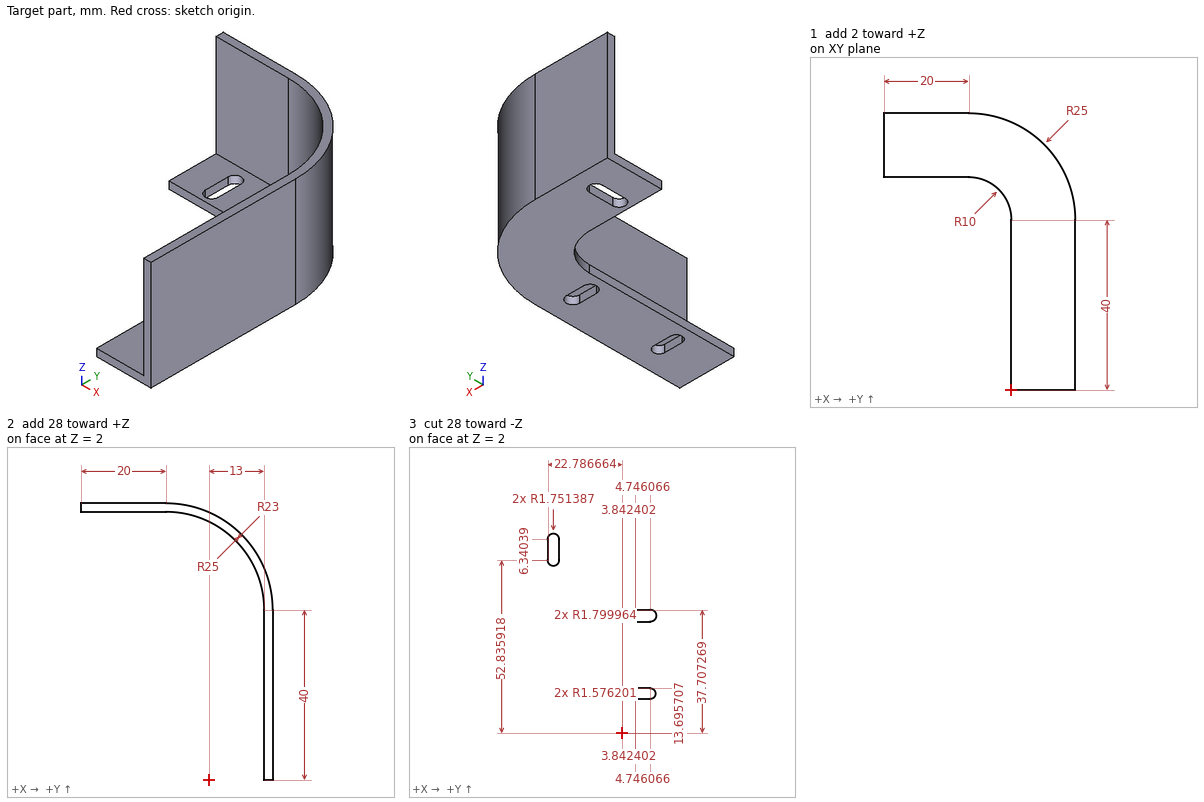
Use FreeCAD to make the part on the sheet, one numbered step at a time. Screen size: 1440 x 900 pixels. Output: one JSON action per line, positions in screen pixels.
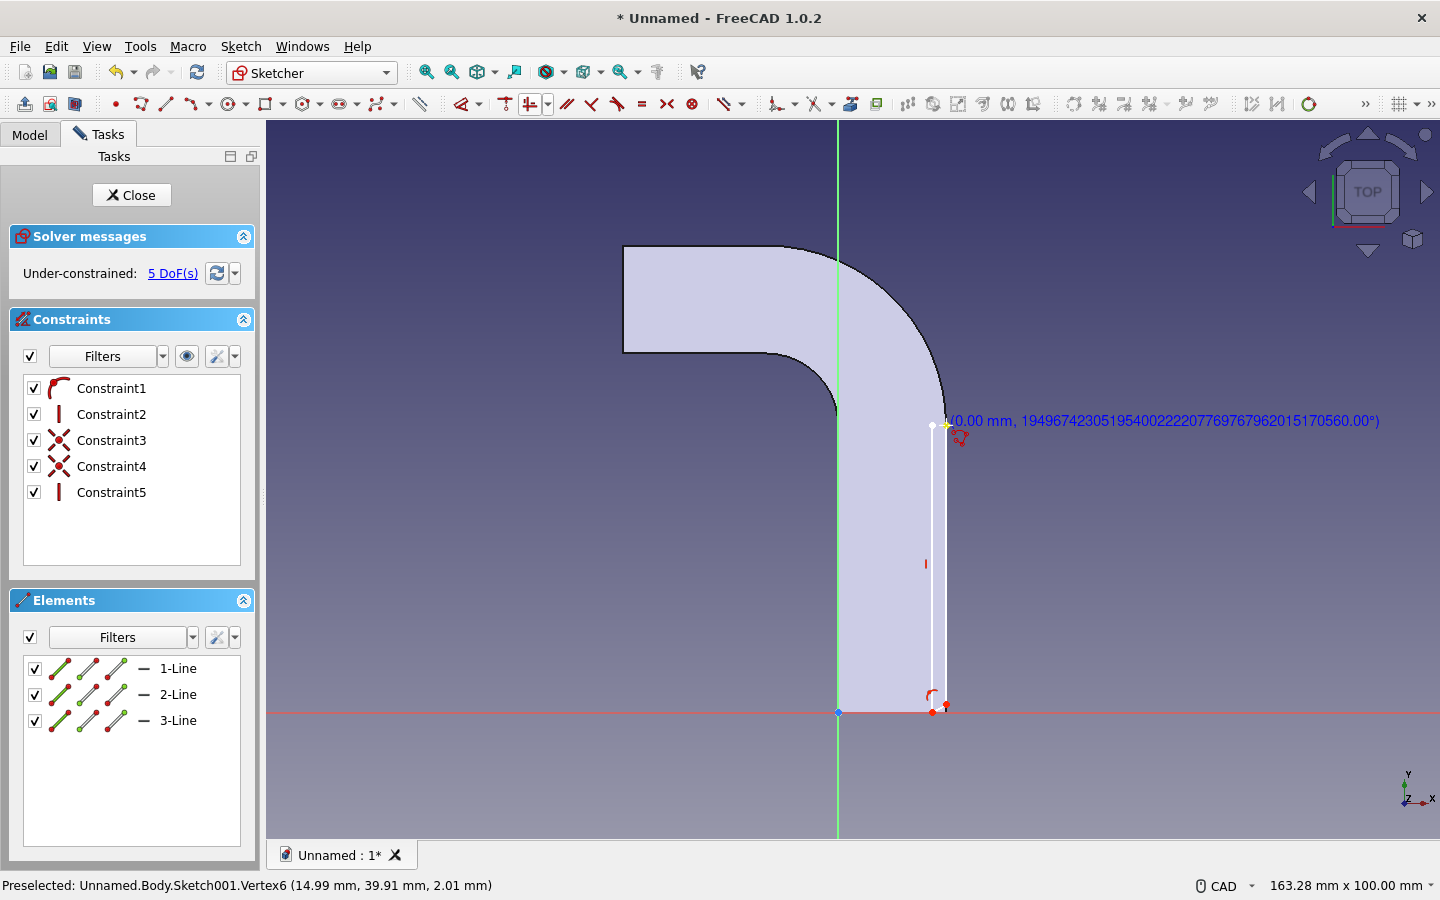
{"action": "left_click", "coordinate": [766, 246]}
{"action": "left_click", "coordinate": [623, 246]}
{"action": "left_click", "coordinate": [623, 260]}
{"action": "left_click", "coordinate": [766, 260]}
{"action": "right_click", "coordinate": [766, 260]}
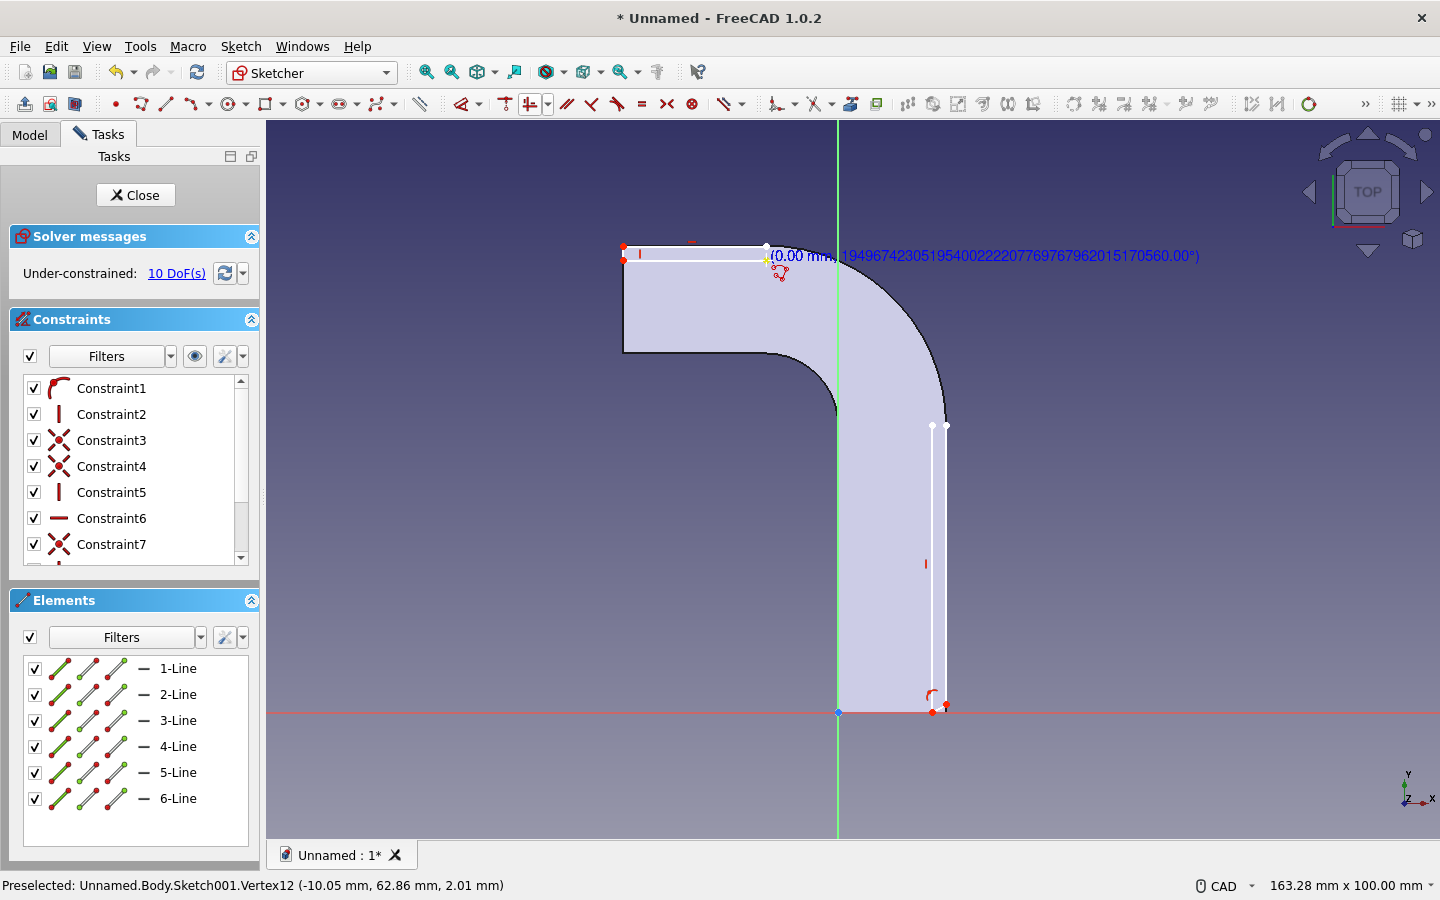
{"action": "left_click", "coordinate": [190, 104]}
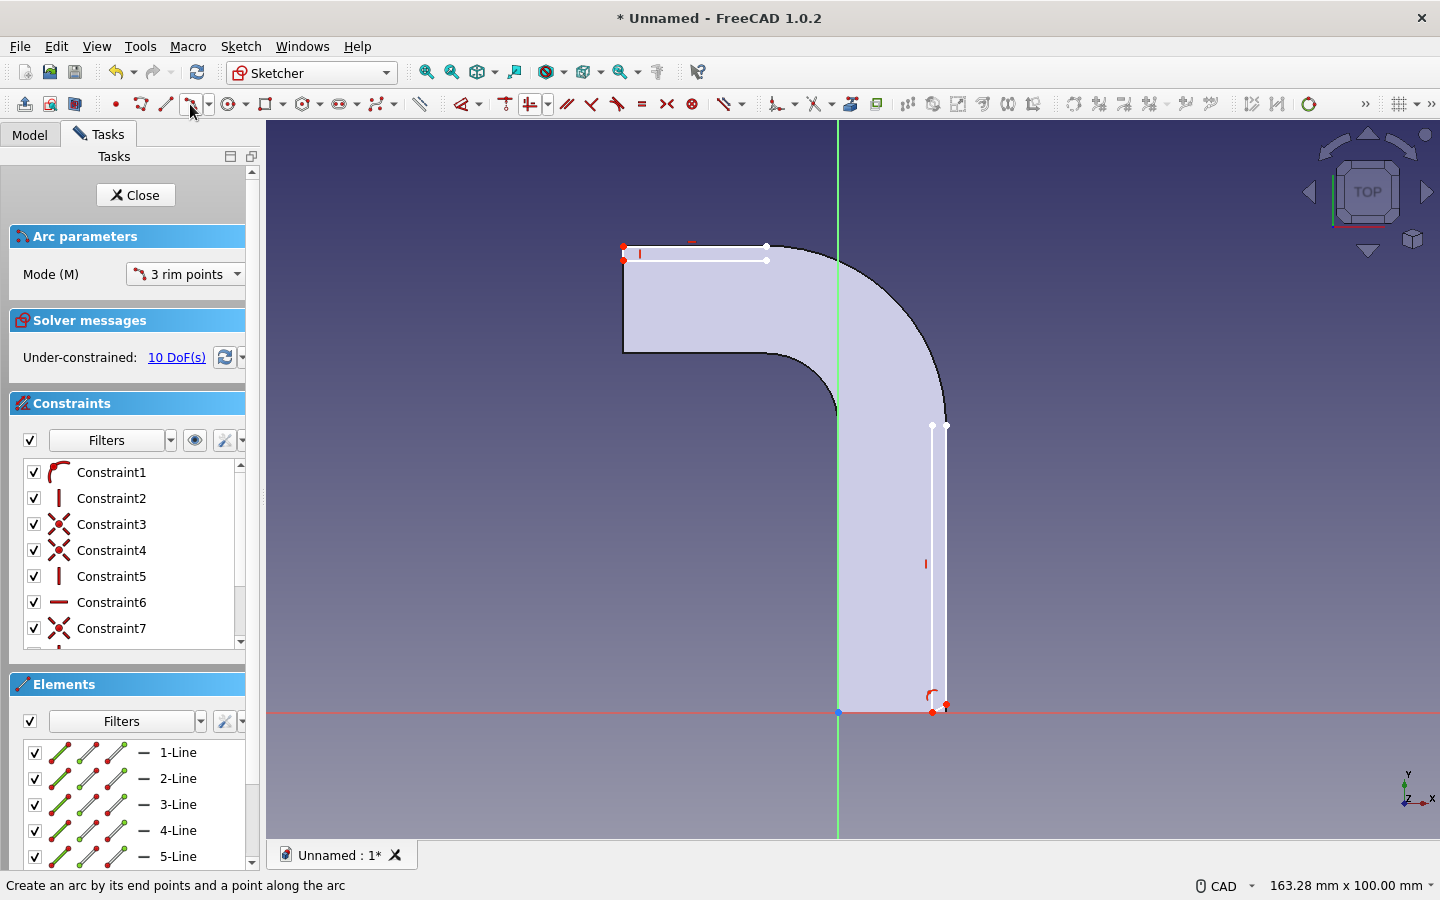
{"action": "left_click", "coordinate": [946, 426]}
{"action": "left_click", "coordinate": [766, 247]}
{"action": "left_click", "coordinate": [893, 298]}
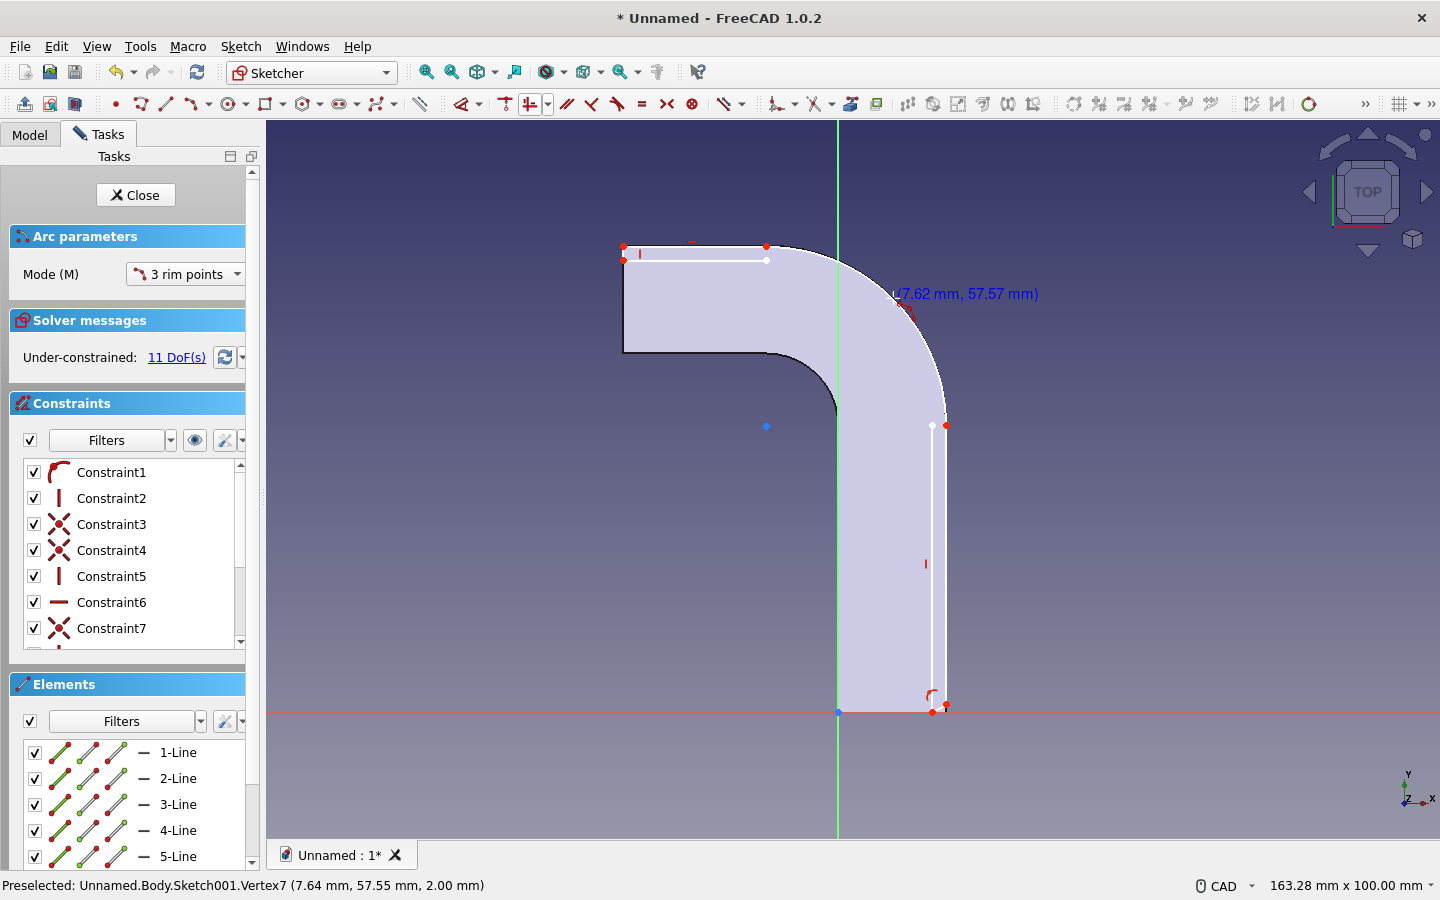
{"action": "left_click", "coordinate": [766, 261]}
{"action": "left_click", "coordinate": [932, 426]}
{"action": "left_click", "coordinate": [883, 308]}
{"action": "key", "text": "Escape"}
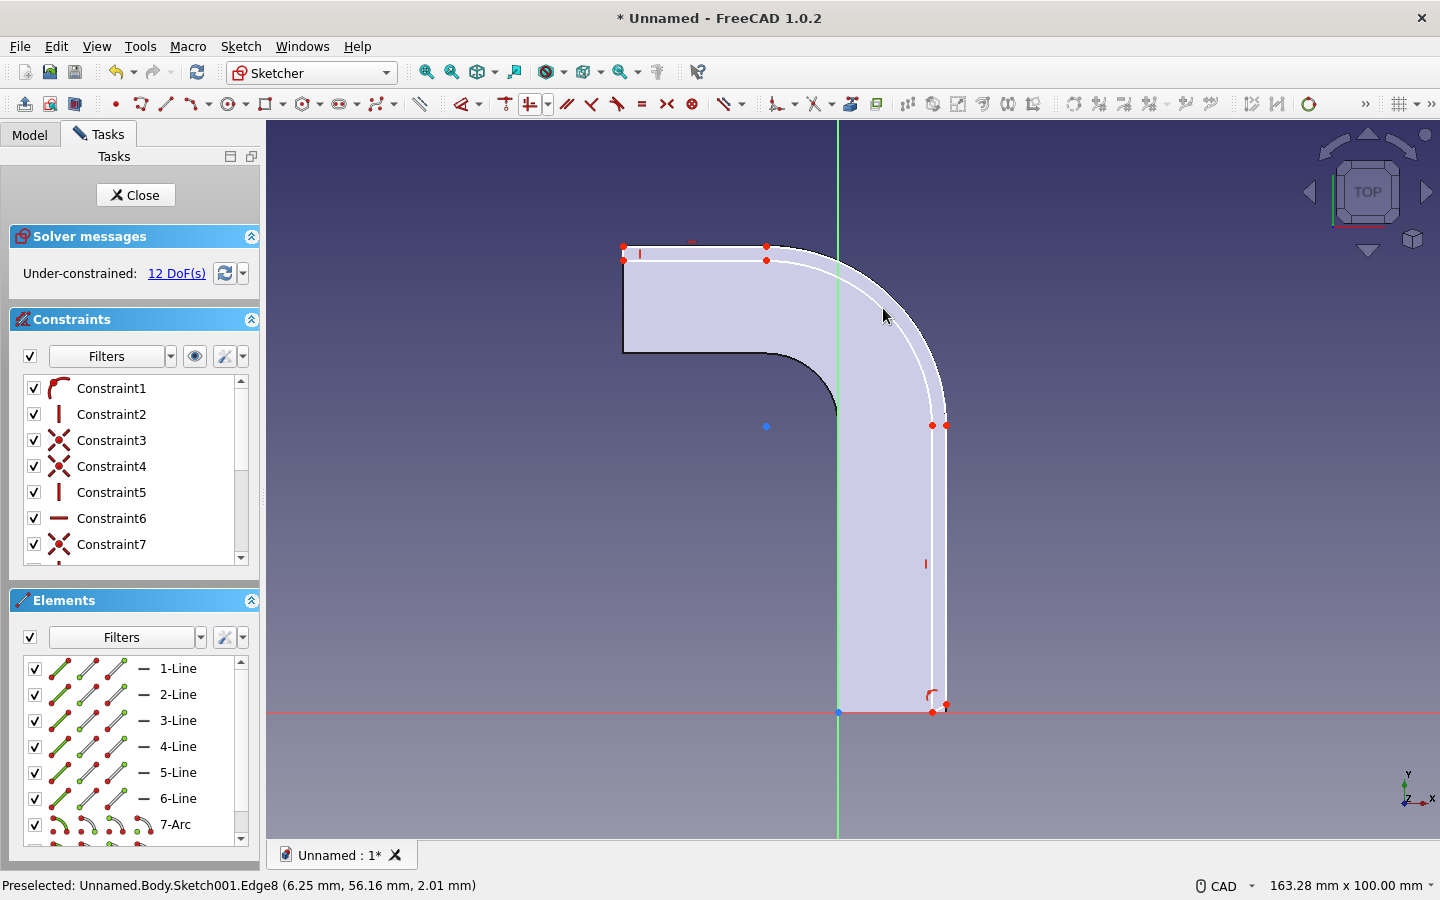
{"action": "left_click", "coordinate": [932, 512]}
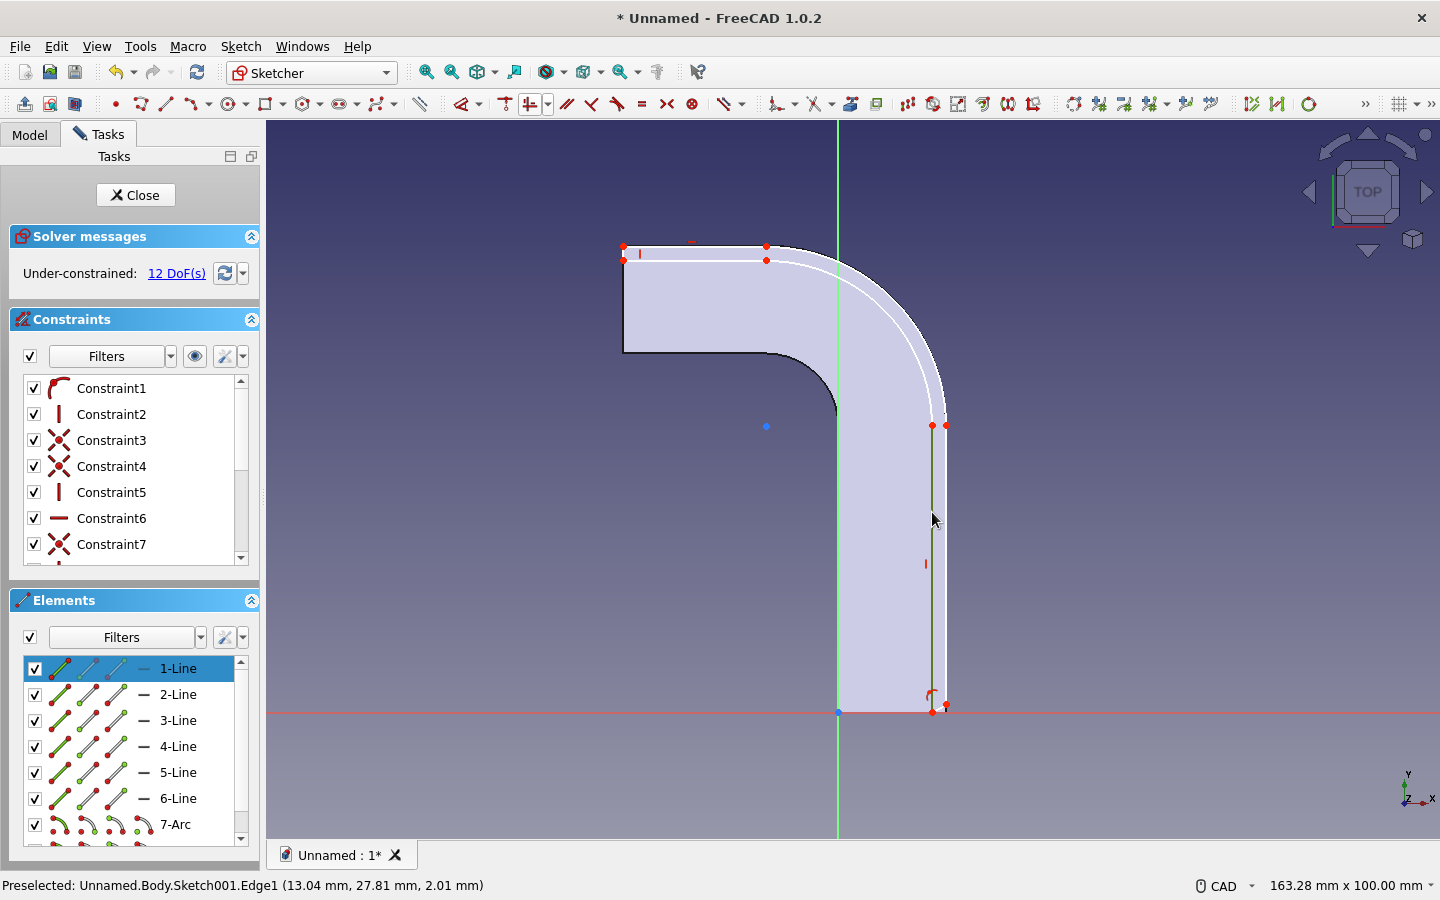
{"action": "left_click", "coordinate": [914, 351]}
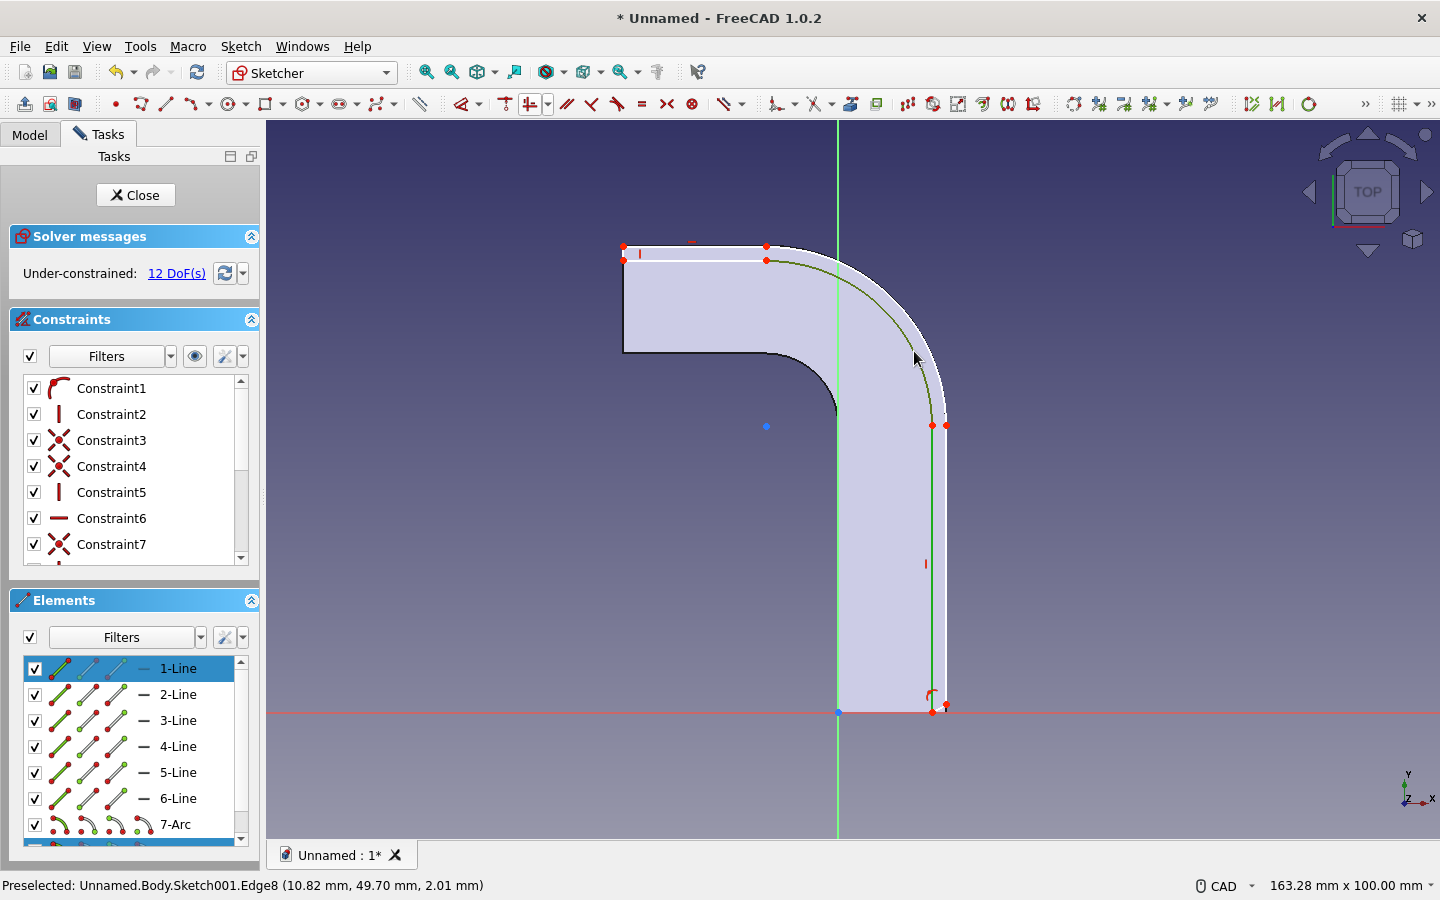
{"action": "left_click", "coordinate": [617, 104]}